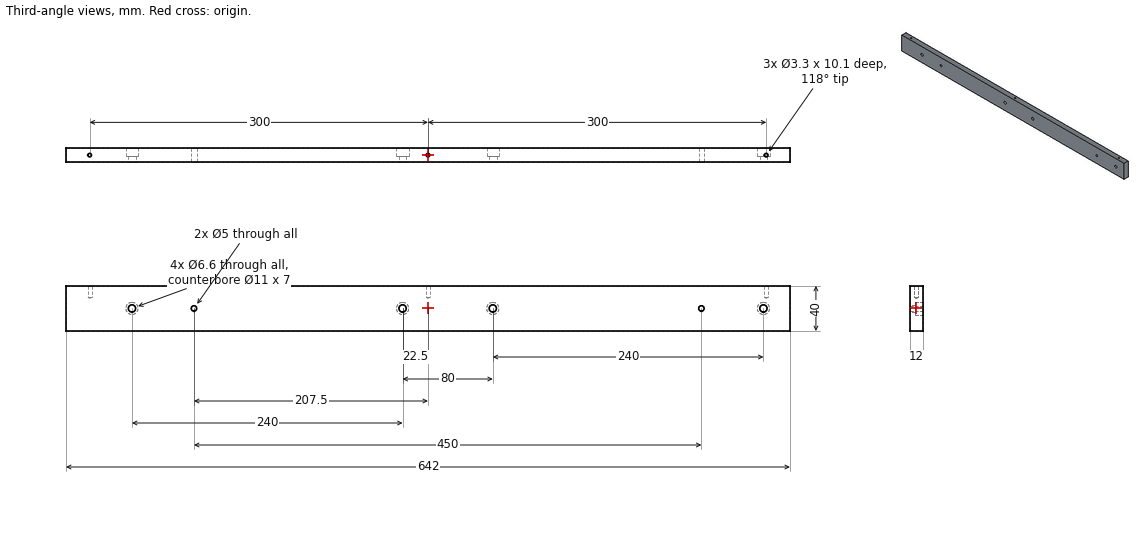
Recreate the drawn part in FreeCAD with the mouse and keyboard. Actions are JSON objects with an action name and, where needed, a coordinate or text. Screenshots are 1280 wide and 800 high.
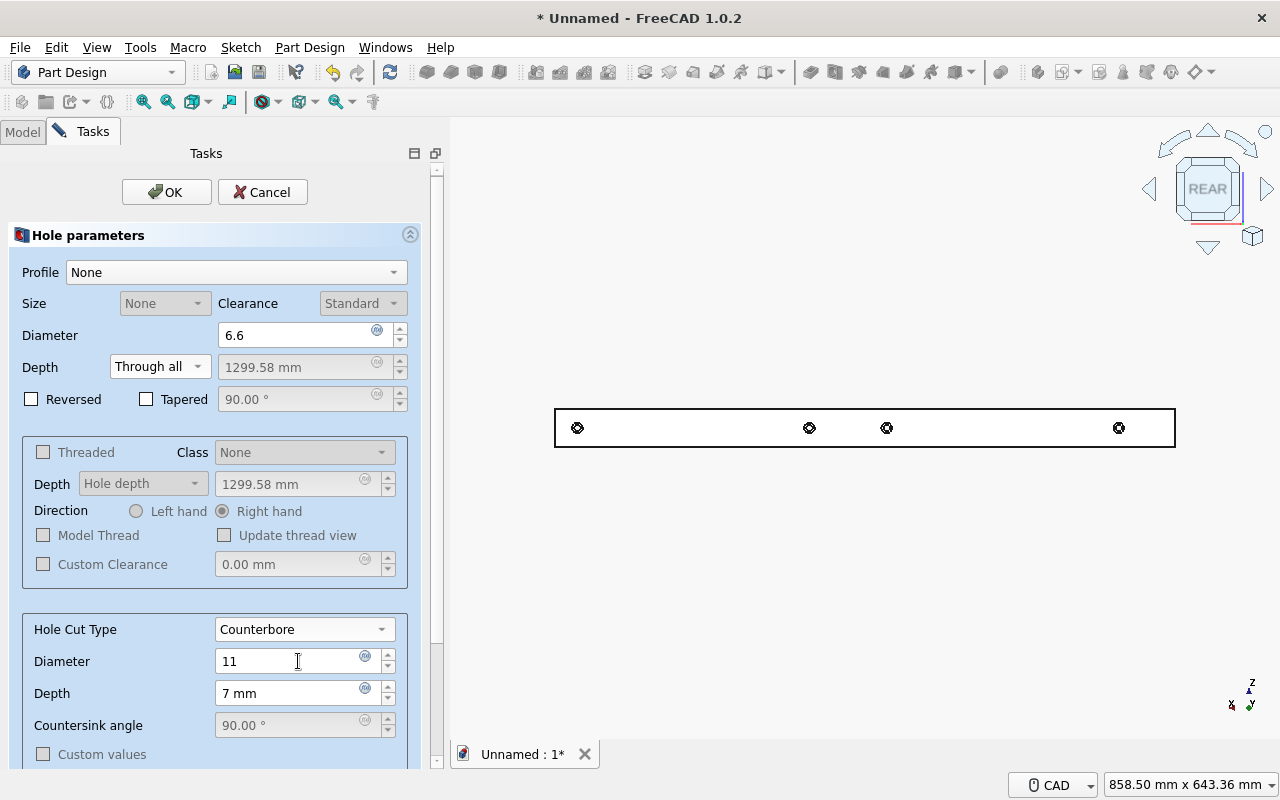
{"action": "left_click", "coordinate": [167, 192]}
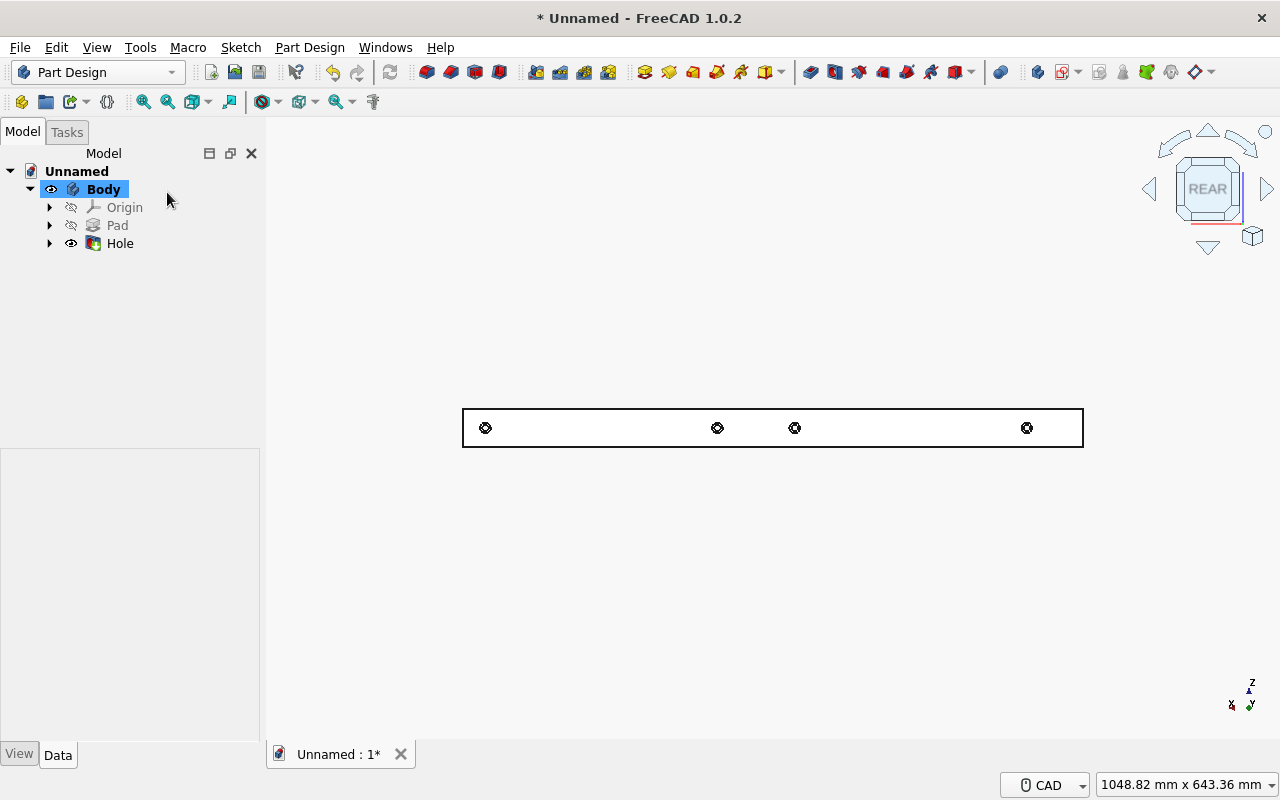
{"action": "key", "text": "0"}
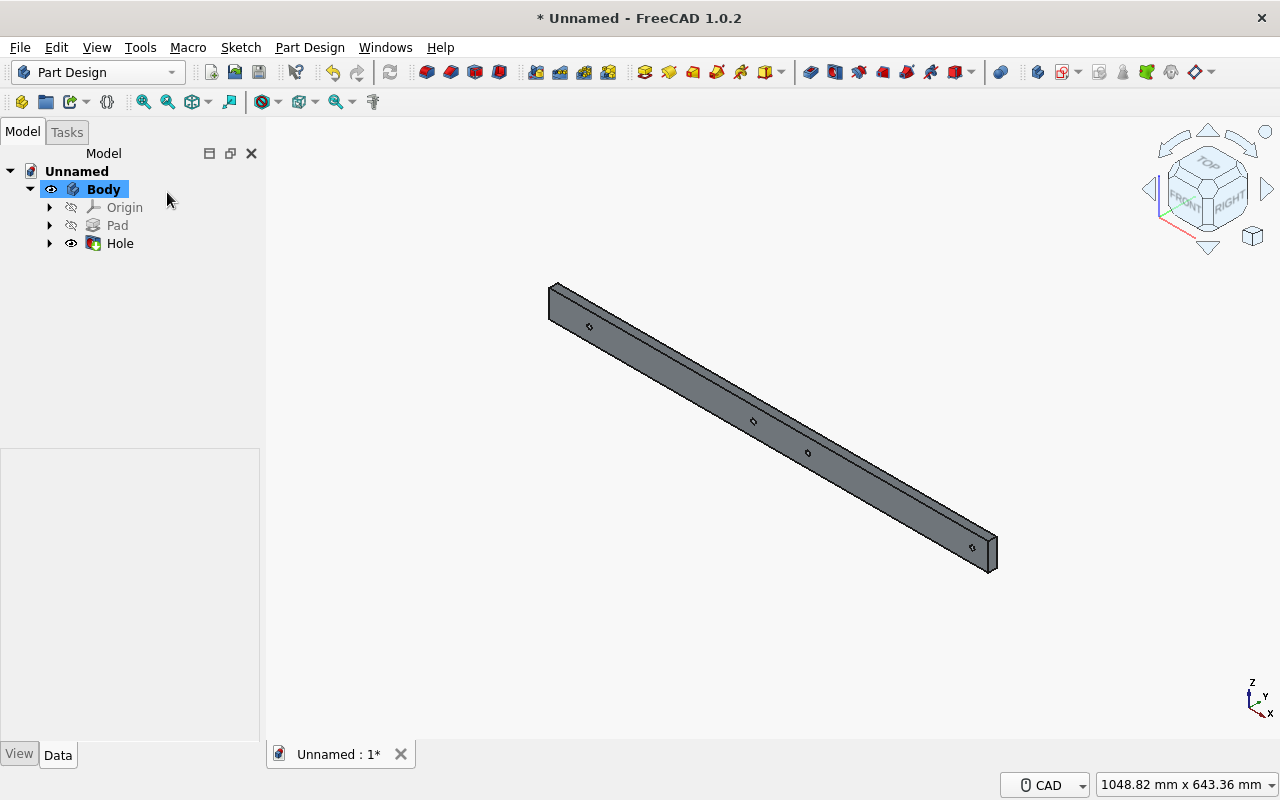
{"action": "scroll", "coordinate": [961, 520], "scroll_direction": "up", "scroll_amount": 4}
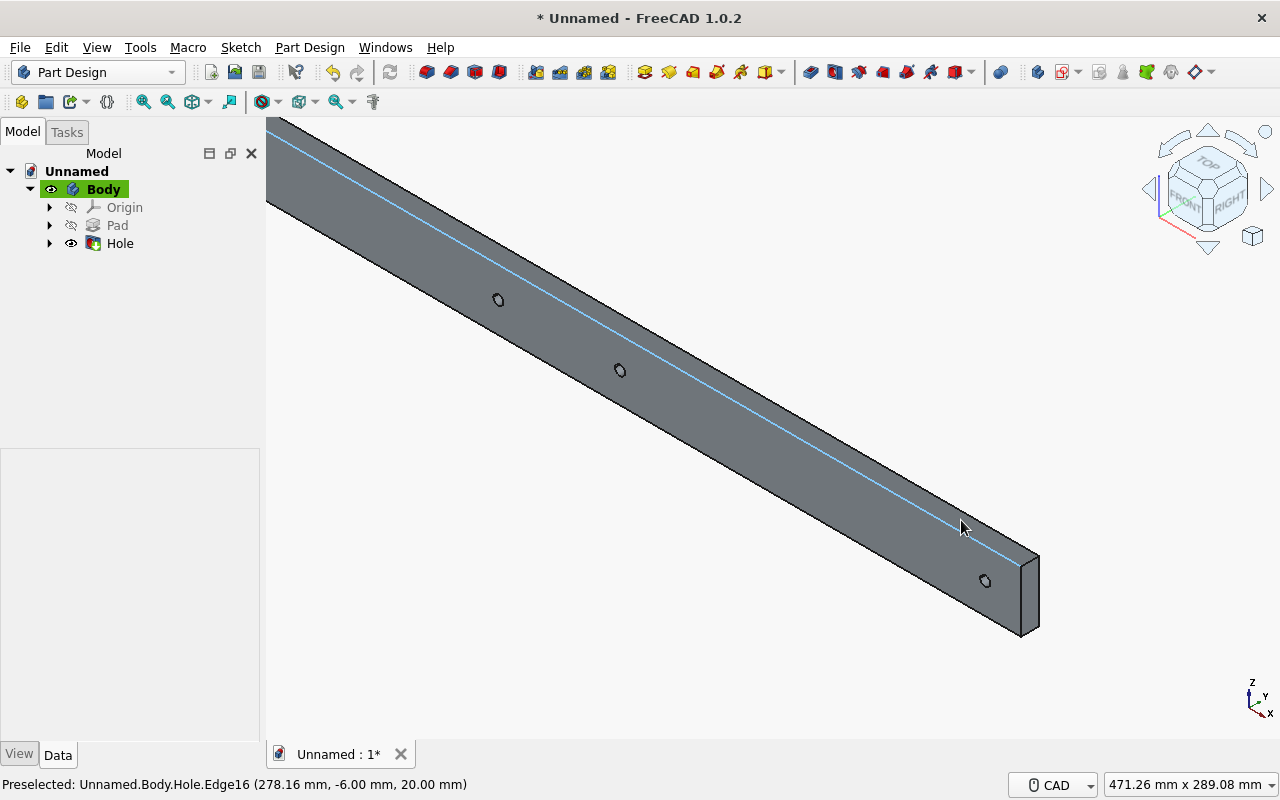
{"action": "left_click", "coordinate": [821, 439]}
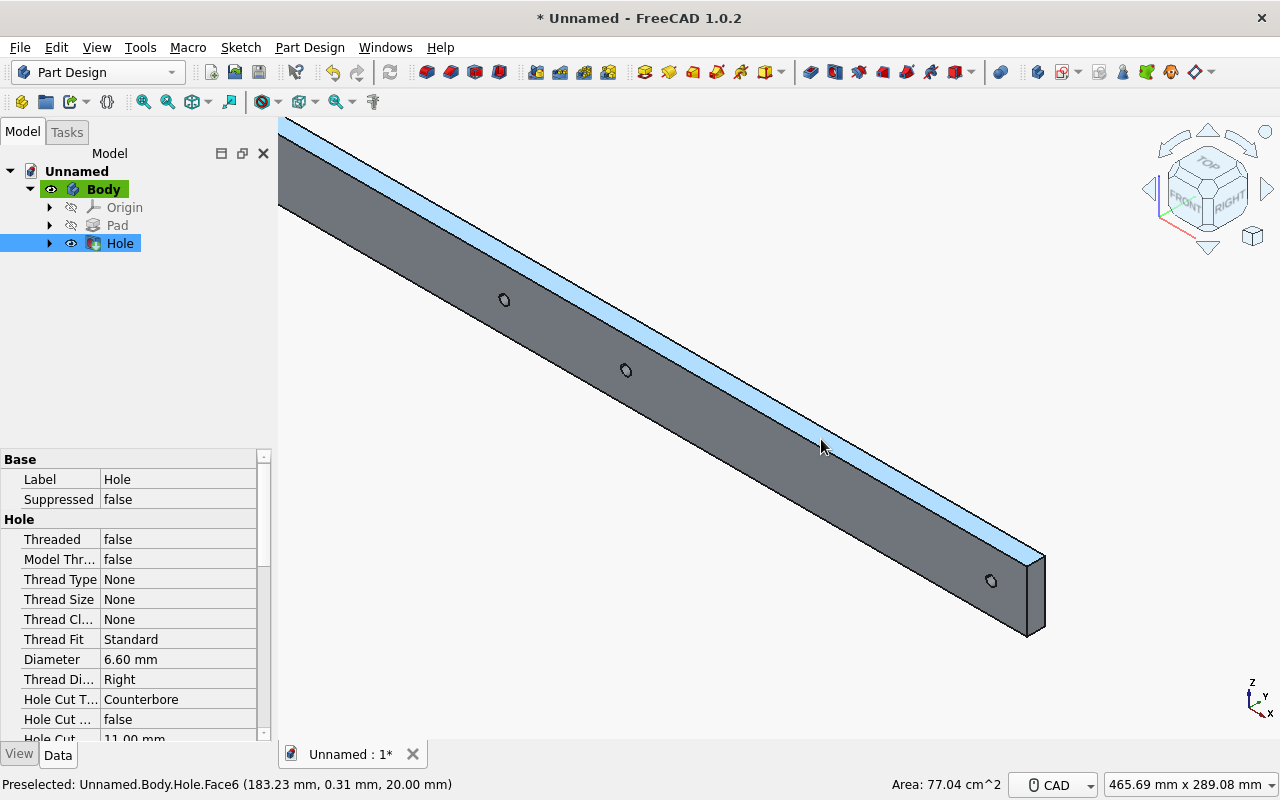
{"action": "left_click", "coordinate": [1062, 72]}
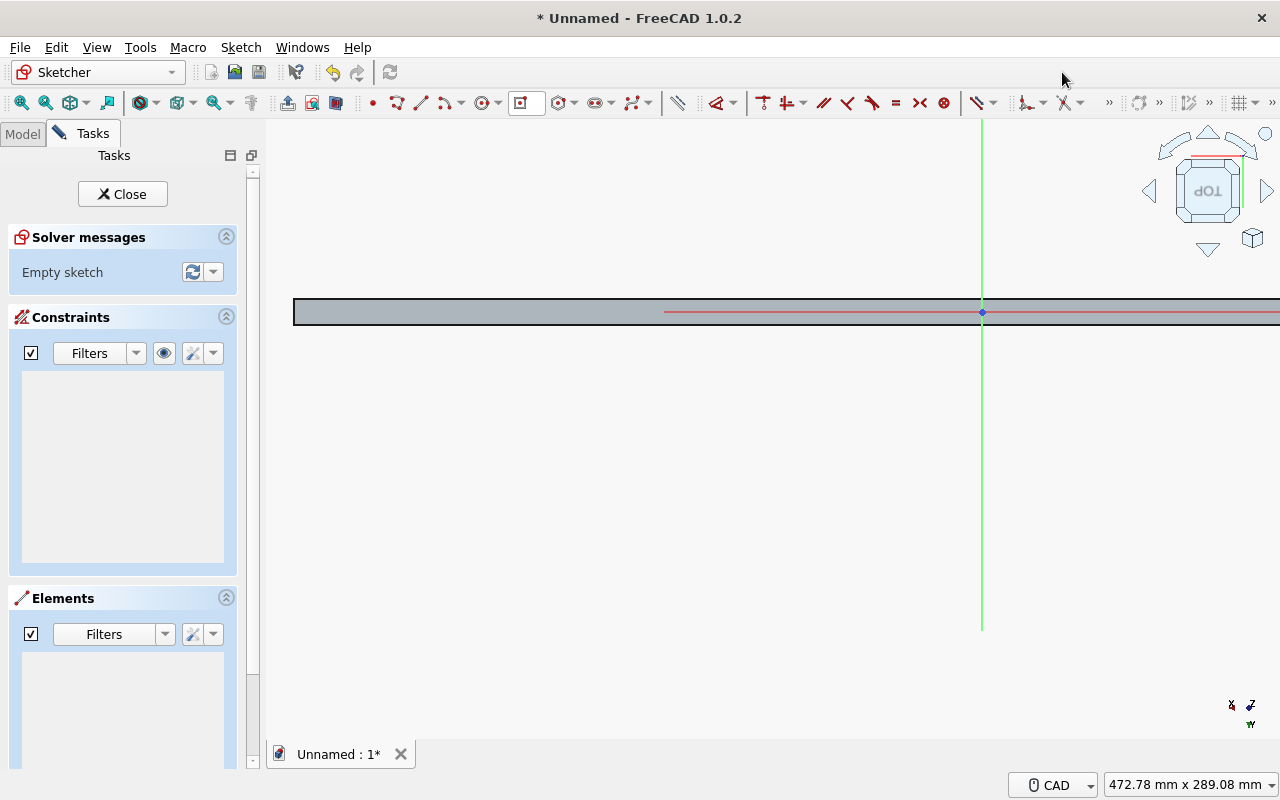
{"action": "scroll", "coordinate": [478, 524], "scroll_direction": "down", "scroll_amount": 4}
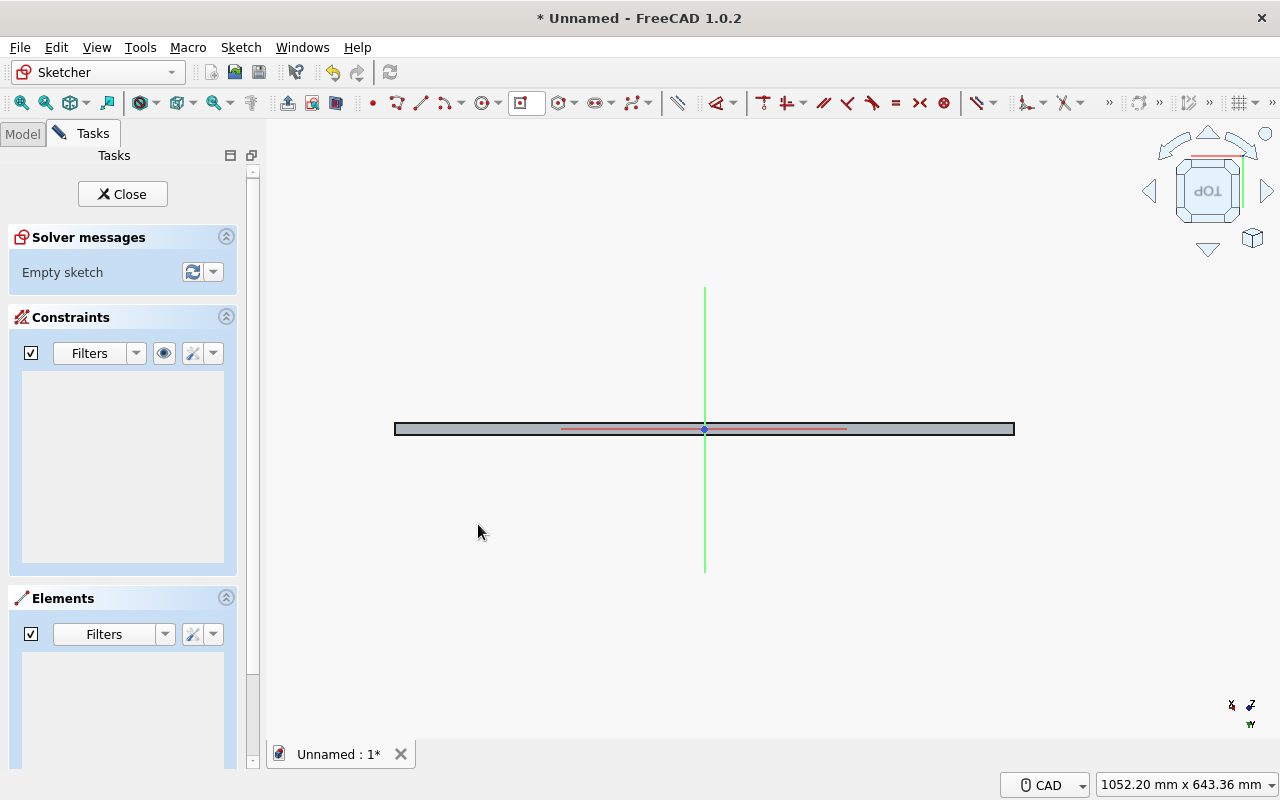
{"action": "left_click", "coordinate": [482, 104]}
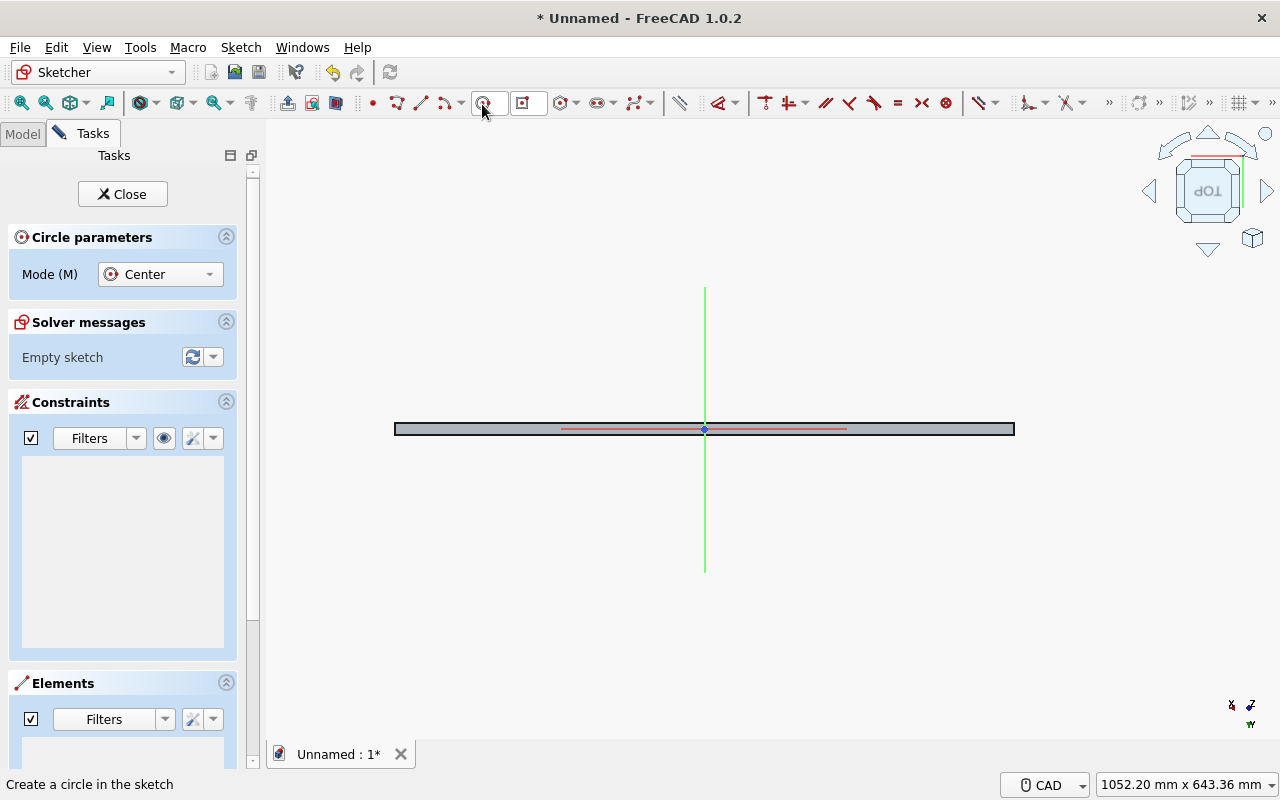
{"action": "scroll", "coordinate": [416, 429], "scroll_direction": "up", "scroll_amount": 14}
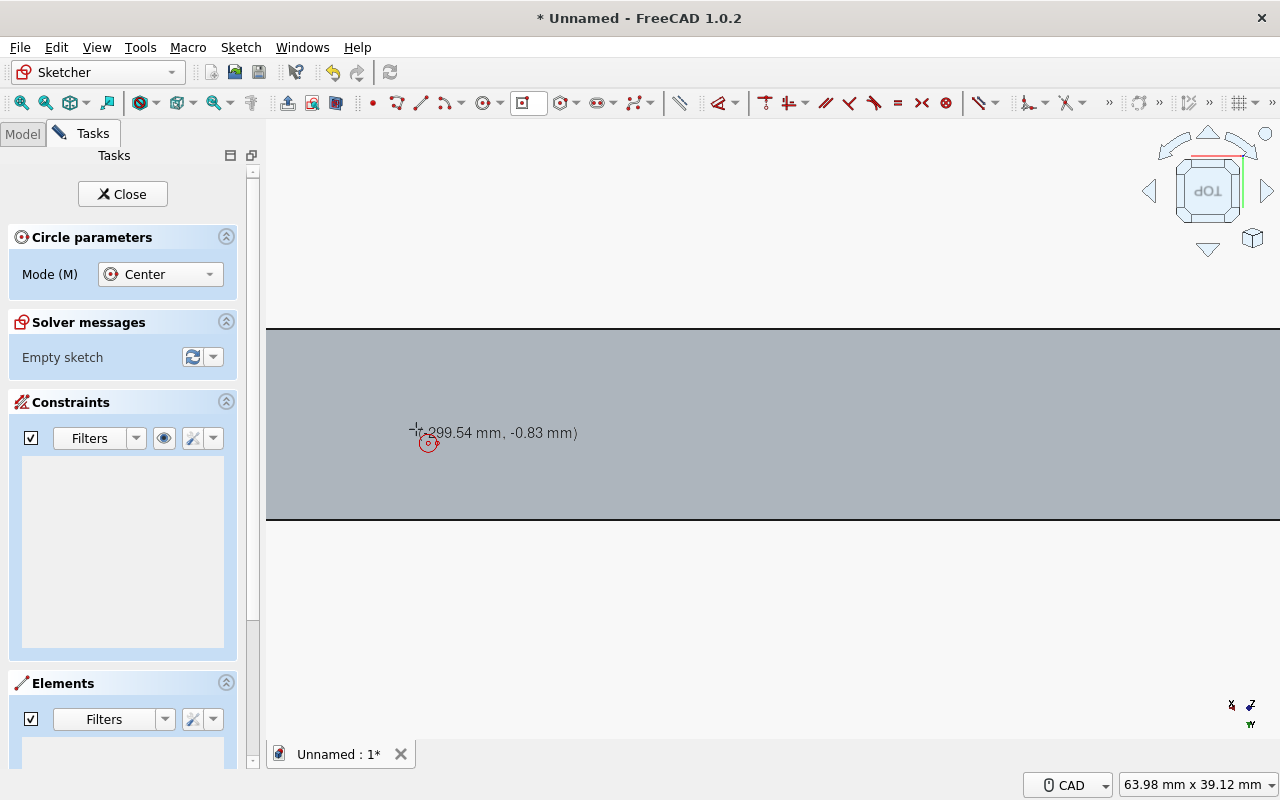
{"action": "scroll", "coordinate": [416, 429], "scroll_direction": "down", "scroll_amount": 14}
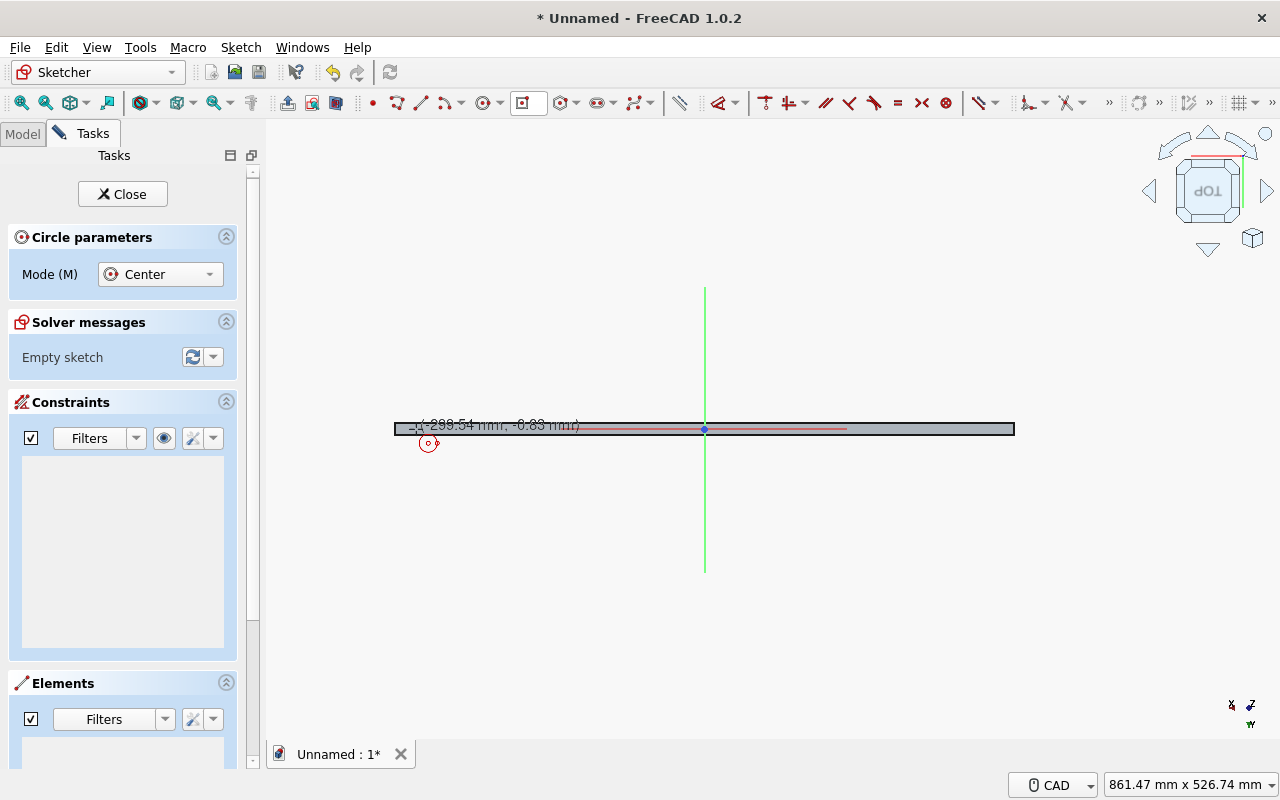
{"action": "left_click", "coordinate": [416, 429]}